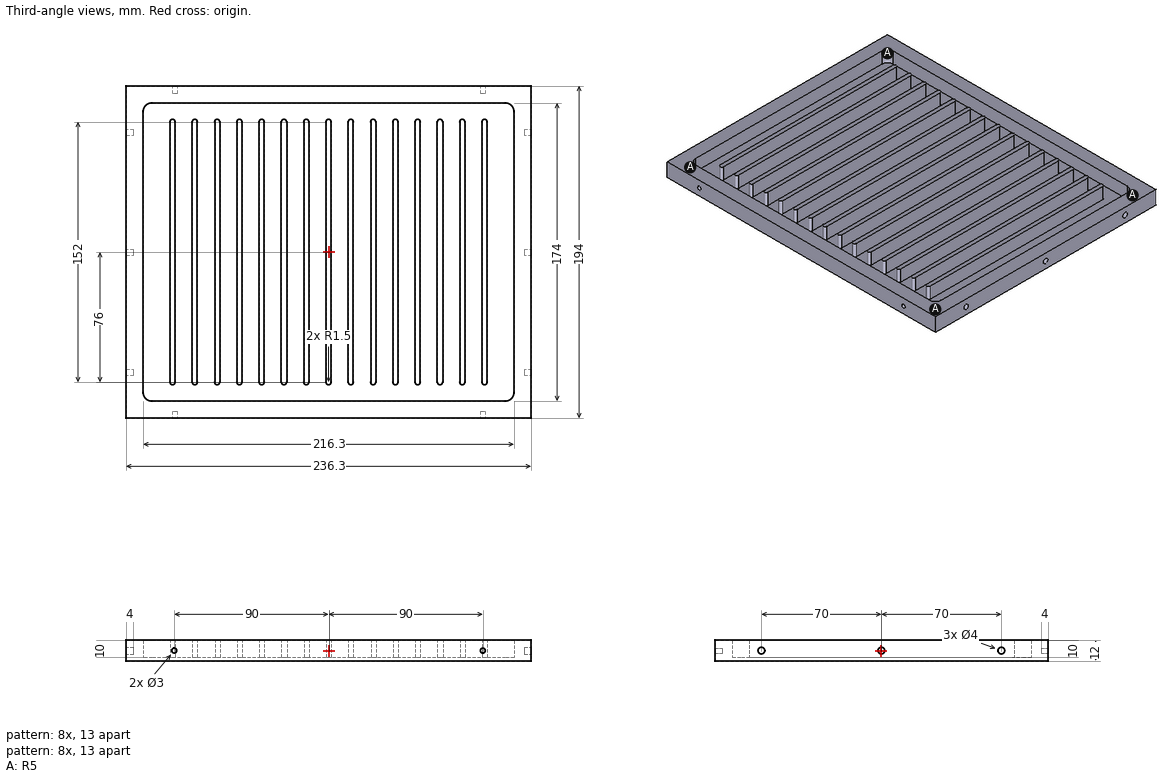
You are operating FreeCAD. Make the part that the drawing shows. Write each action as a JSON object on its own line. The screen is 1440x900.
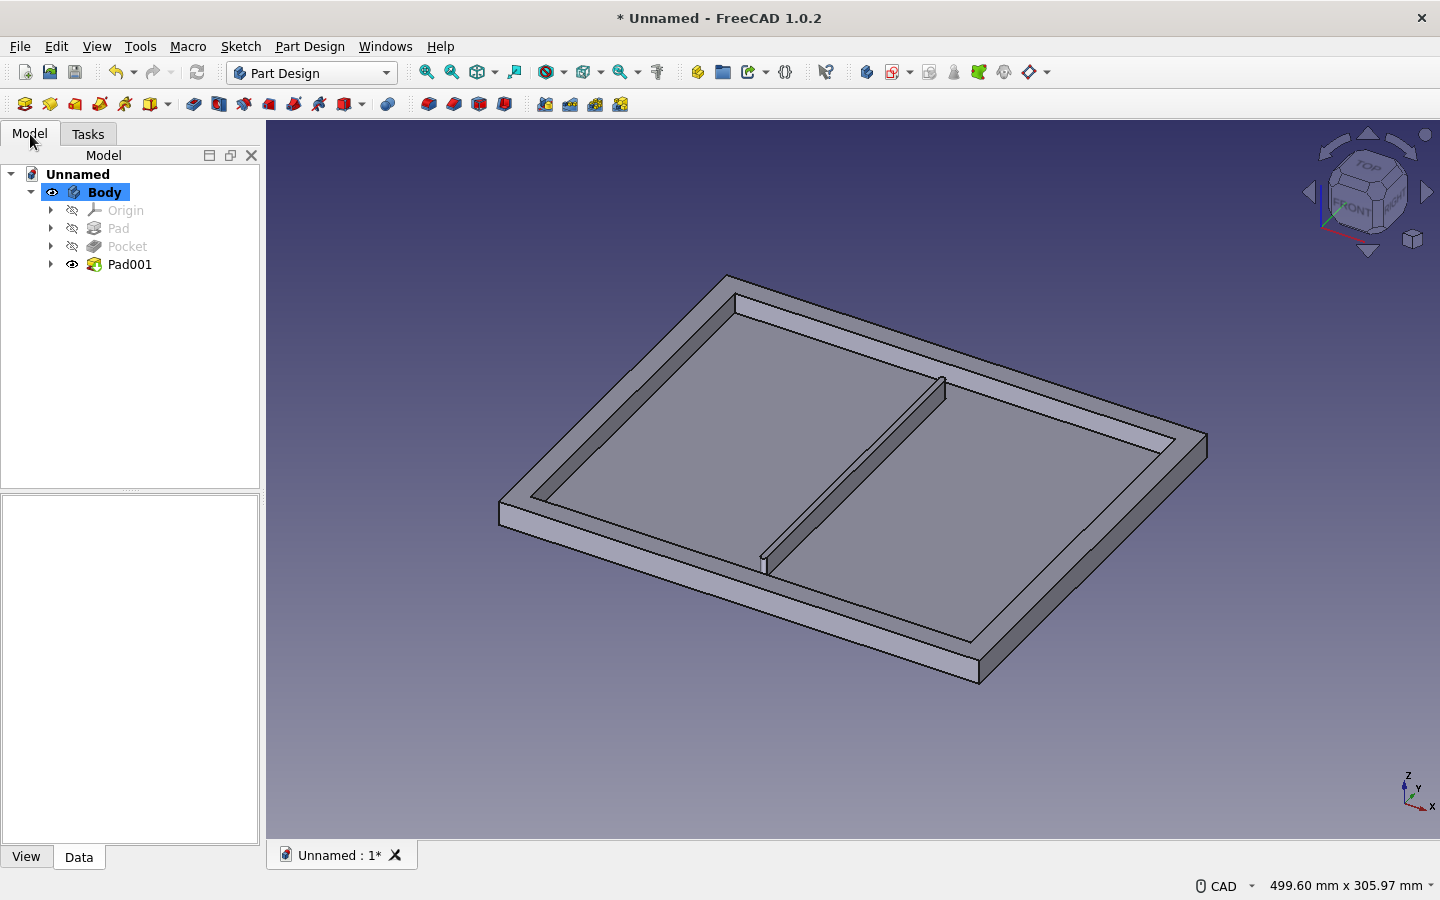
{"action": "left_click", "coordinate": [117, 264]}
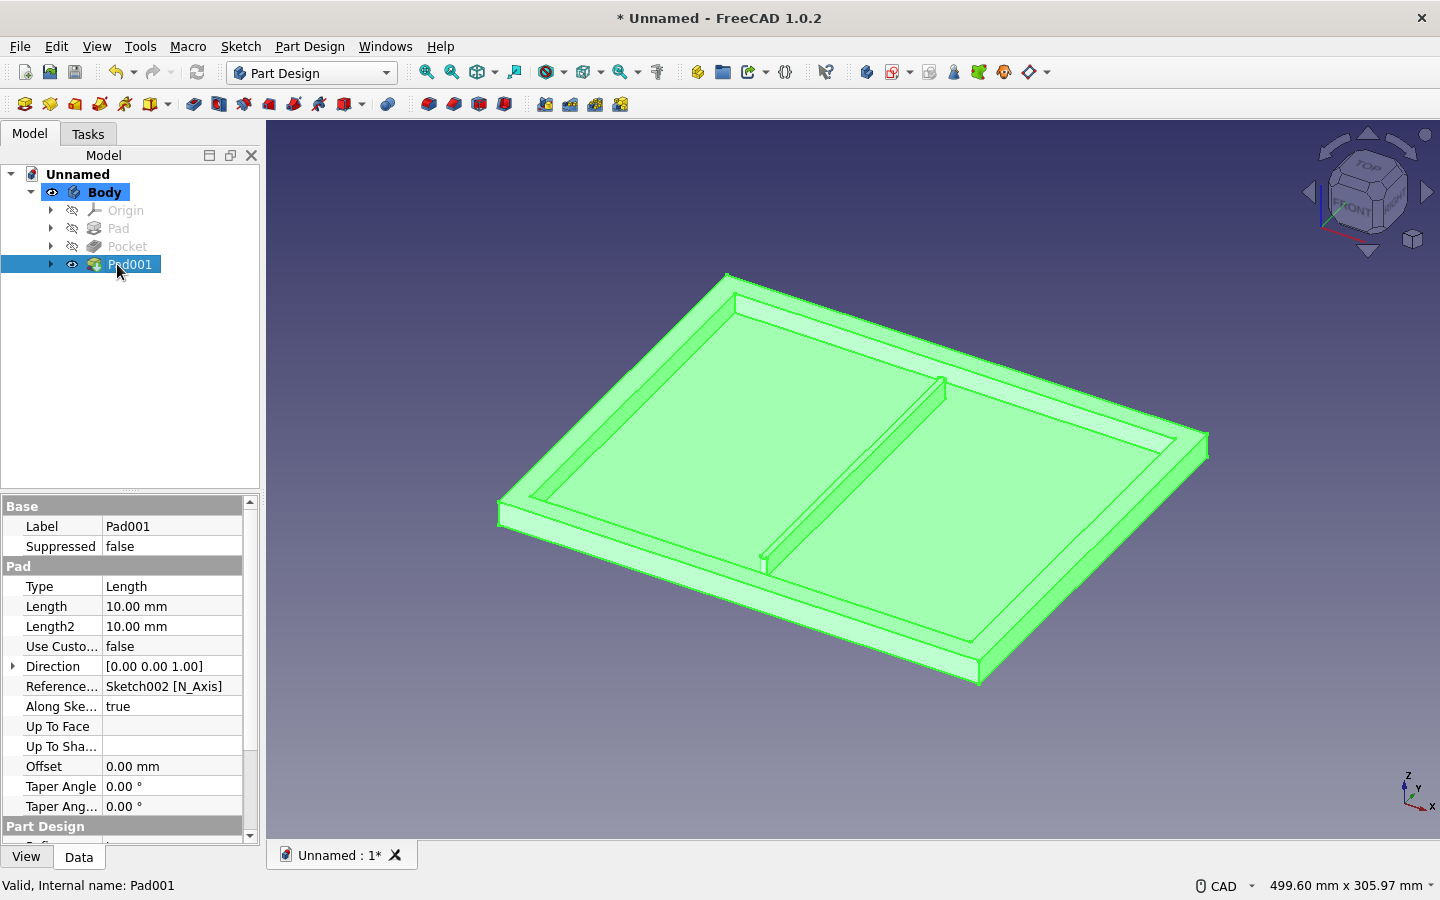
{"action": "left_click", "coordinate": [570, 104]}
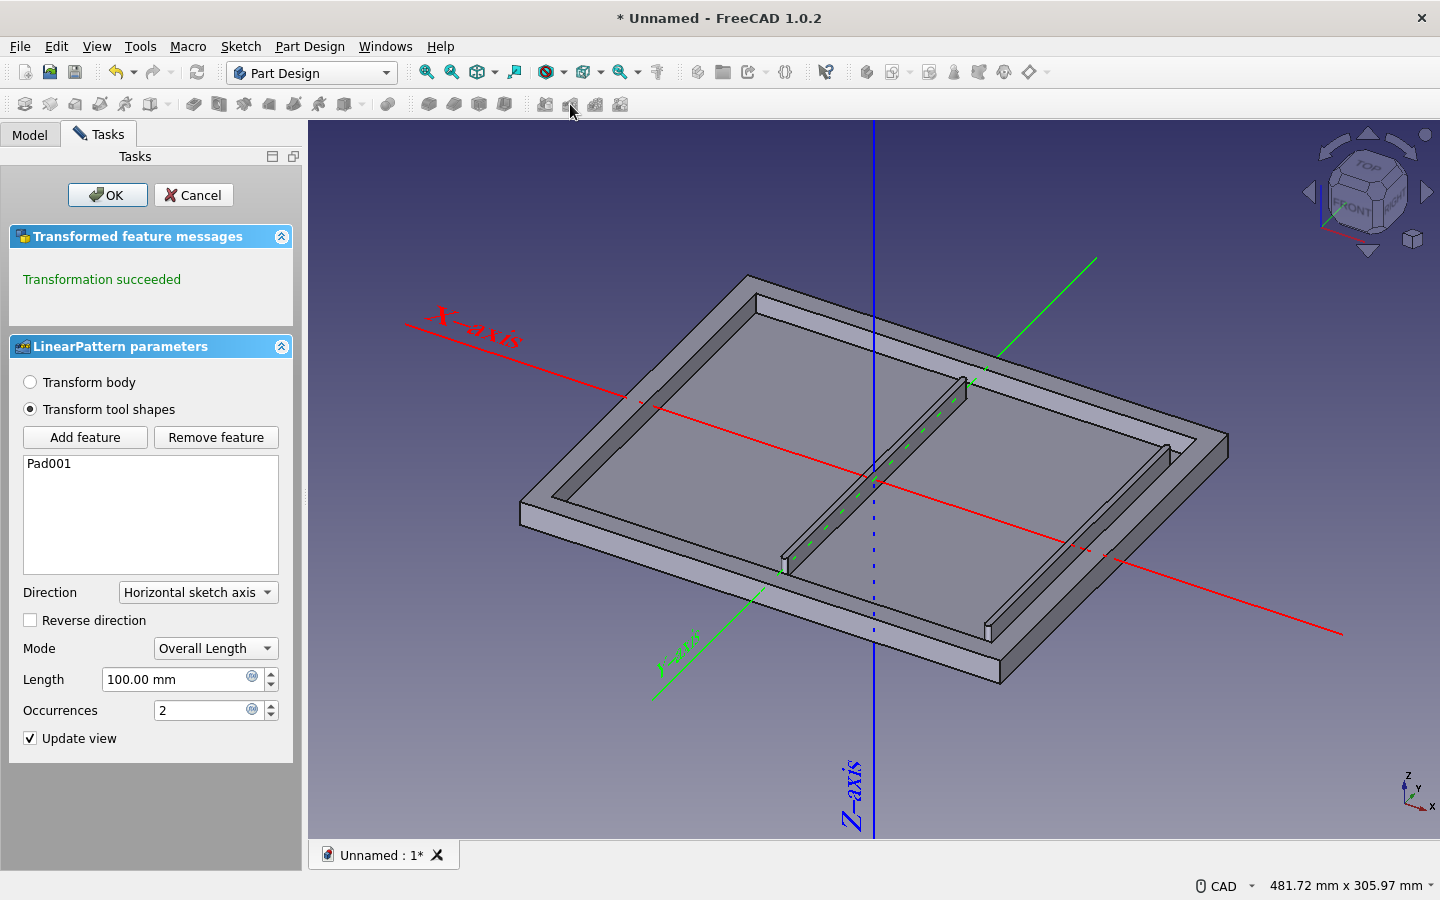
{"action": "left_click", "coordinate": [199, 592]}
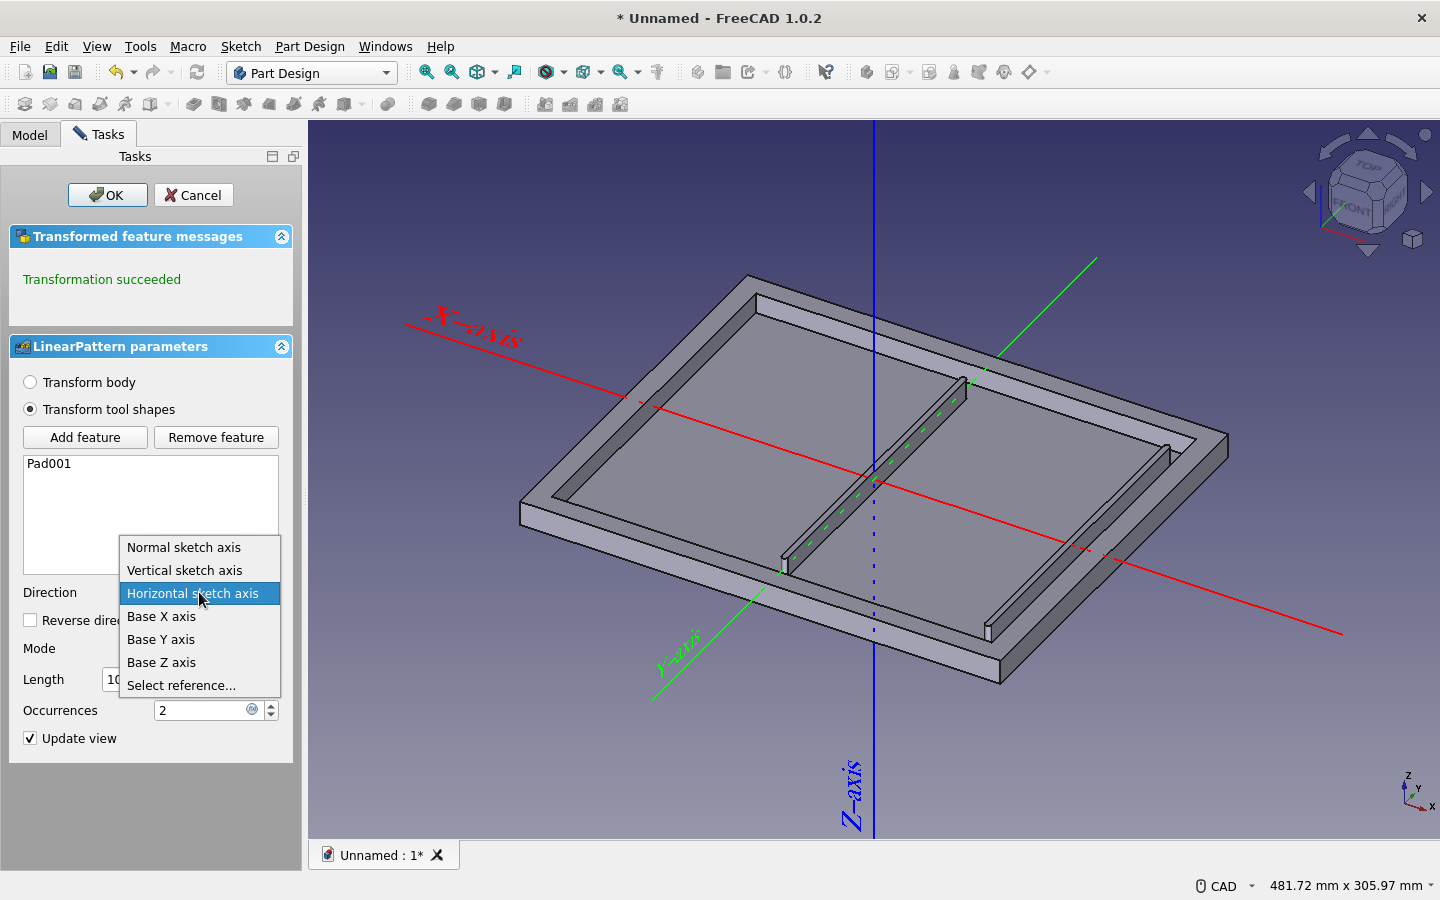
{"action": "left_click", "coordinate": [198, 616]}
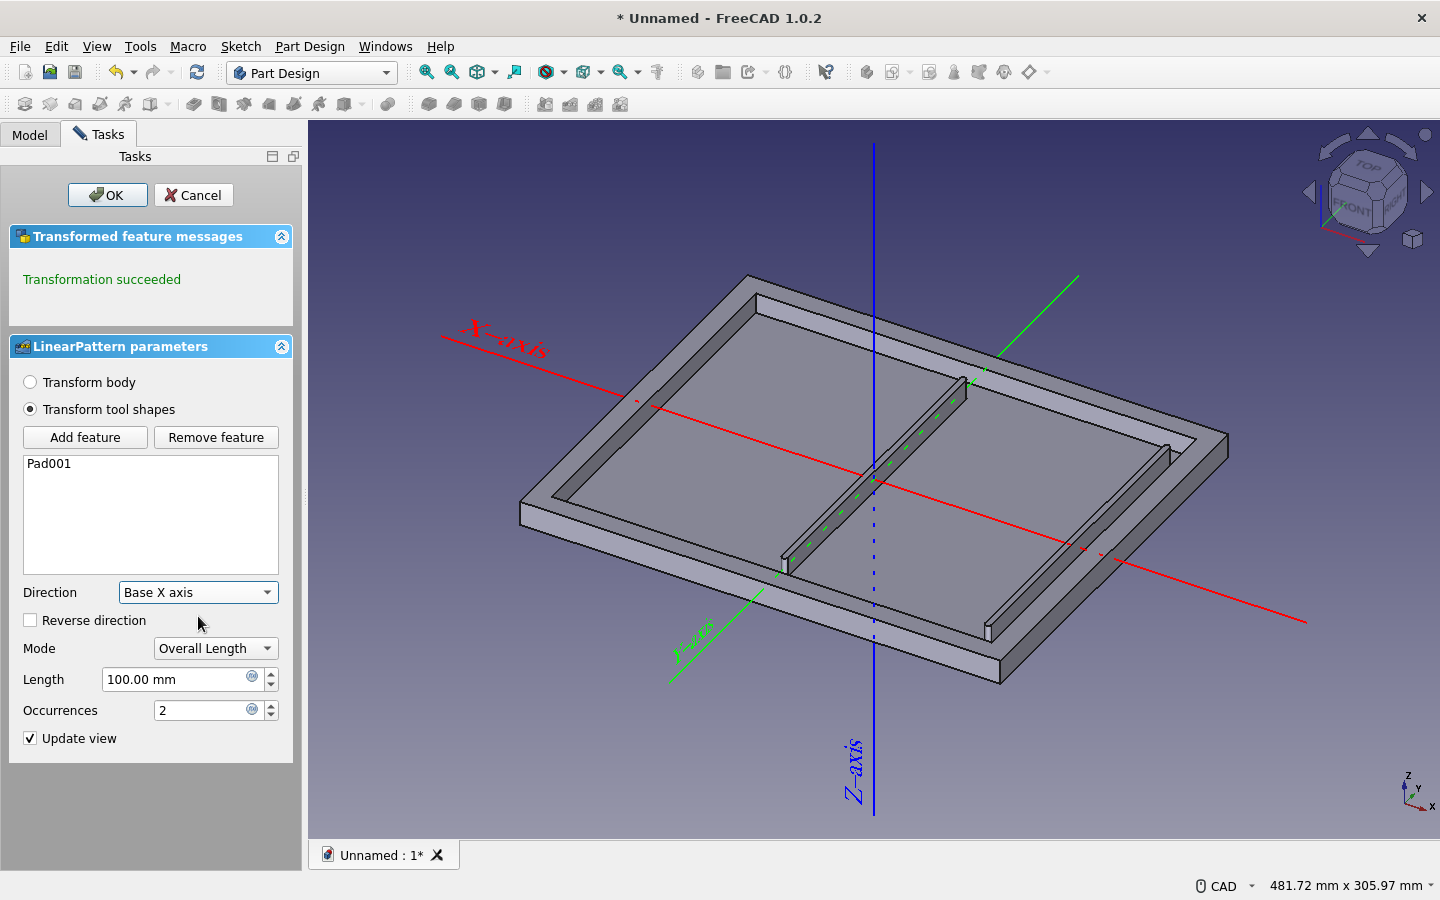
{"action": "left_click", "coordinate": [216, 648]}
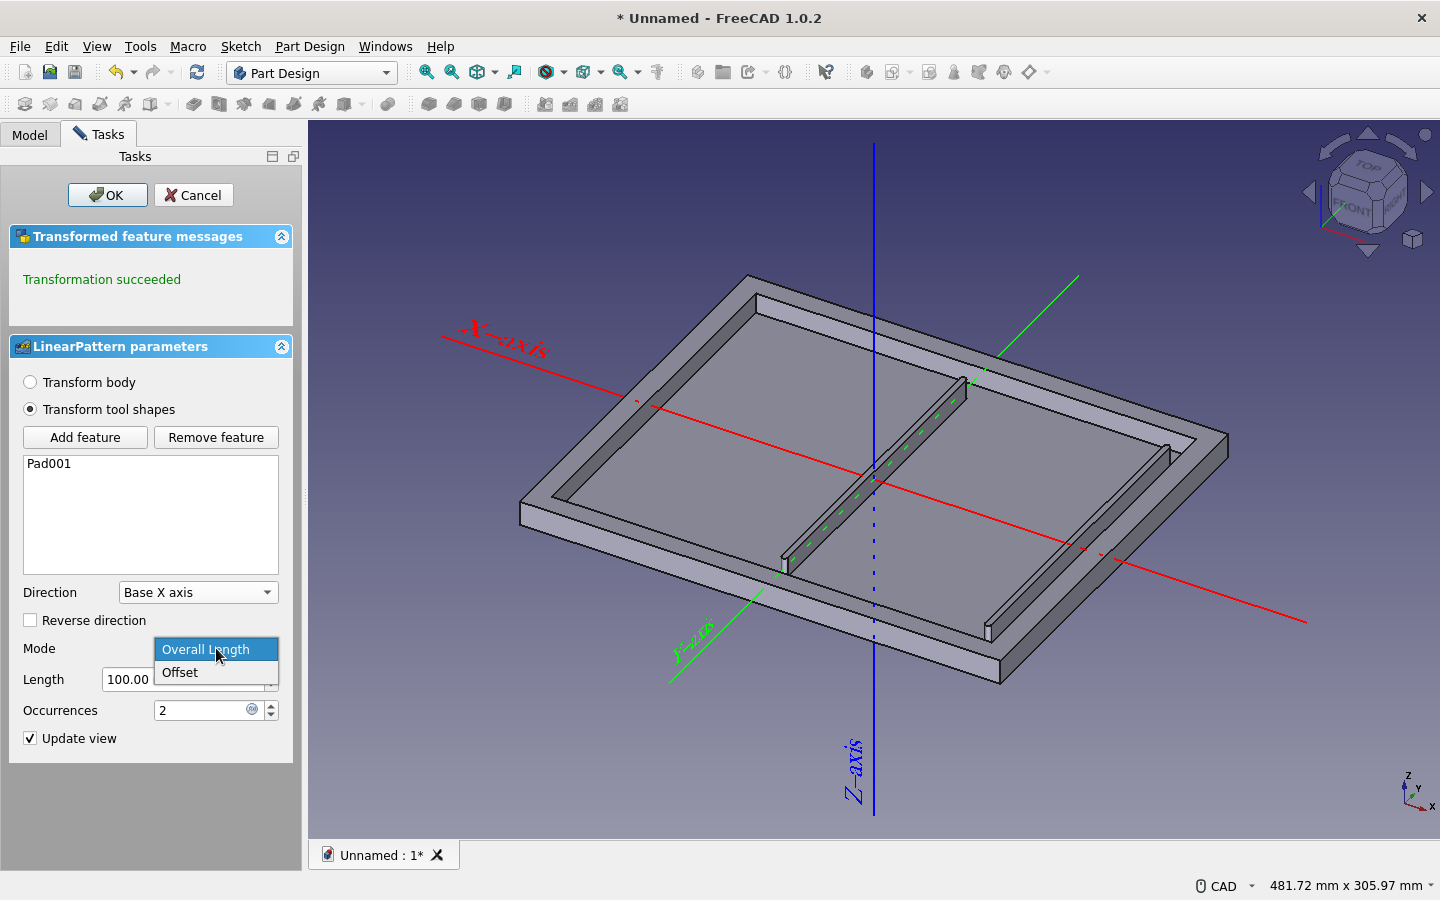
{"action": "left_click", "coordinate": [214, 672]}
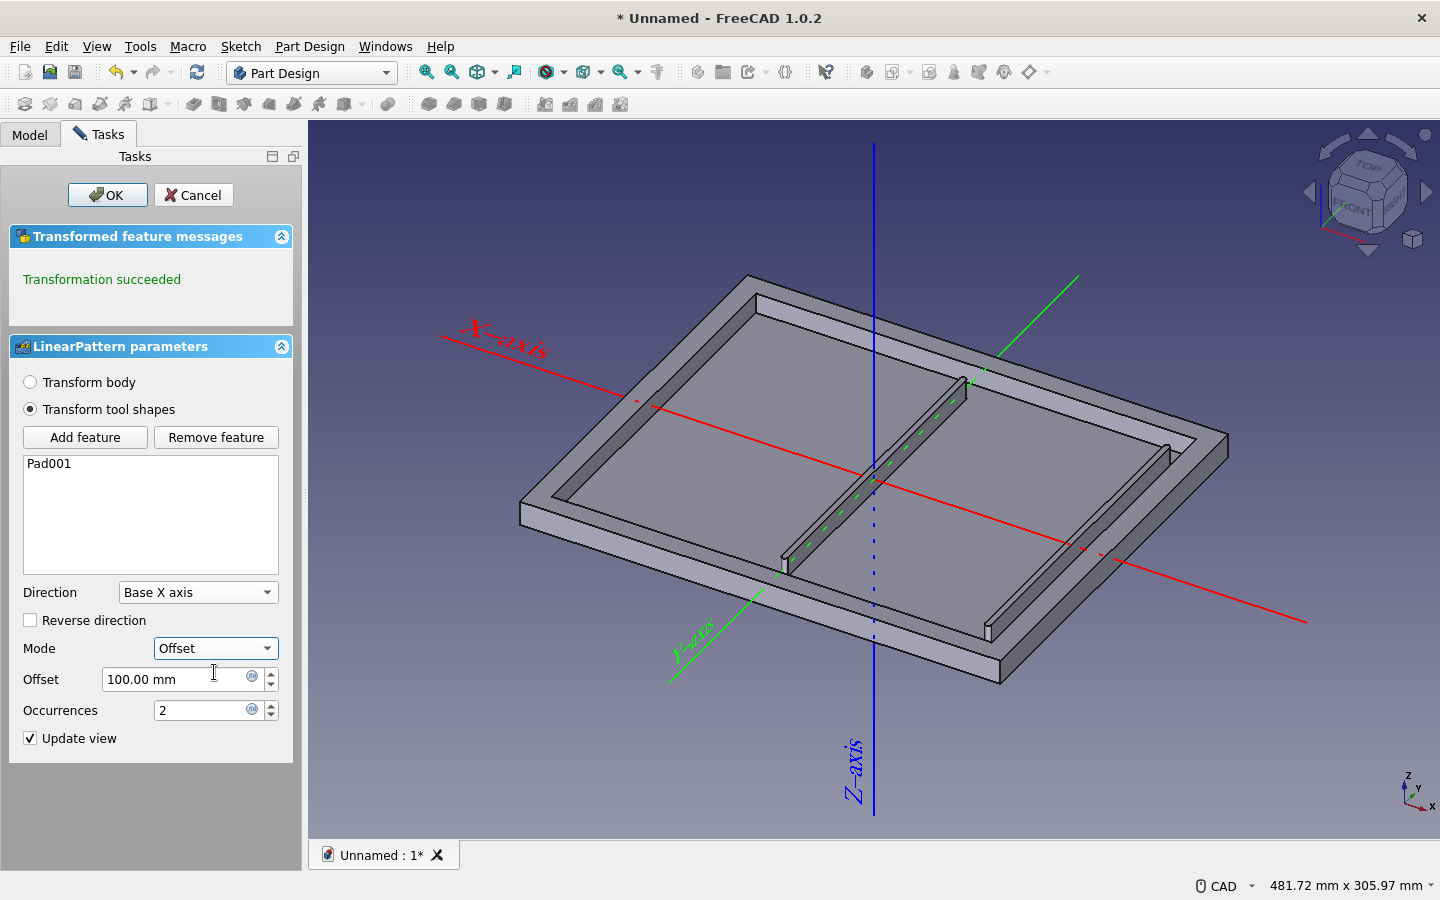
{"action": "triple_click", "coordinate": [184, 680]}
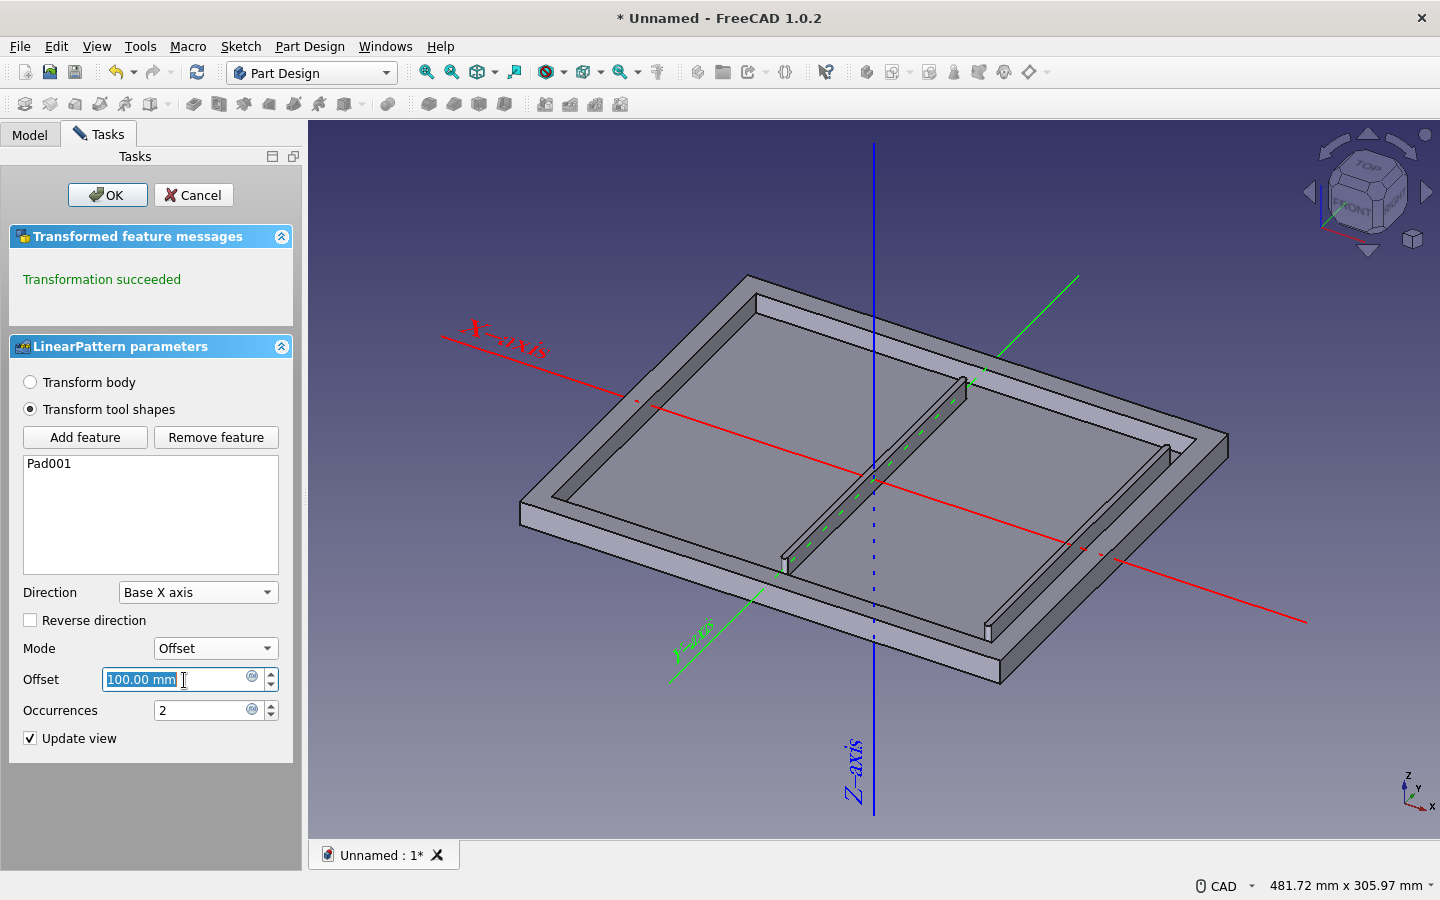
{"action": "type", "text": "13"}
{"action": "key", "text": "Tab"}